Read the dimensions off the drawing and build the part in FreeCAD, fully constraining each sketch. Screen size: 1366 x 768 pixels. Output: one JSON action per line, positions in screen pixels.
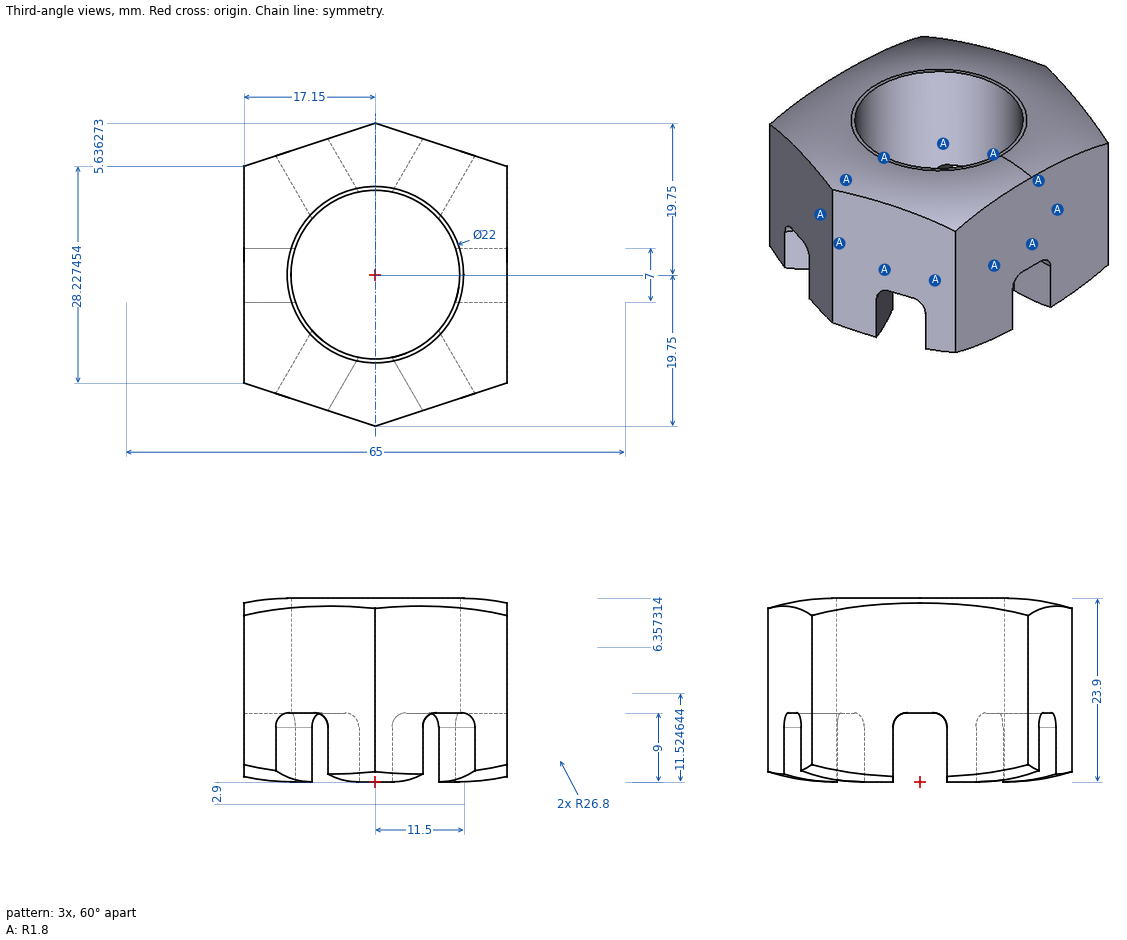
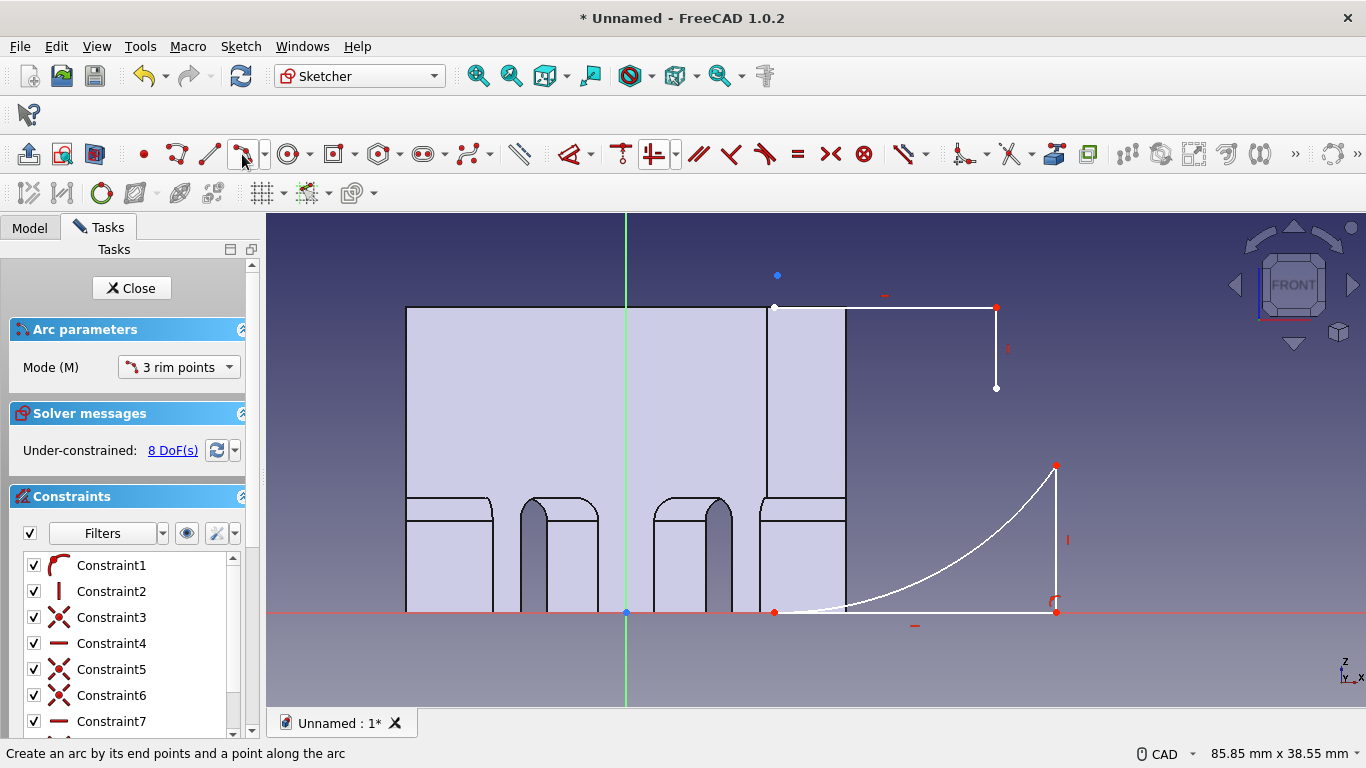
{"action": "left_click", "coordinate": [996, 389]}
{"action": "left_click", "coordinate": [774, 308]}
{"action": "left_click", "coordinate": [892, 328]}
{"action": "key", "text": "Escape"}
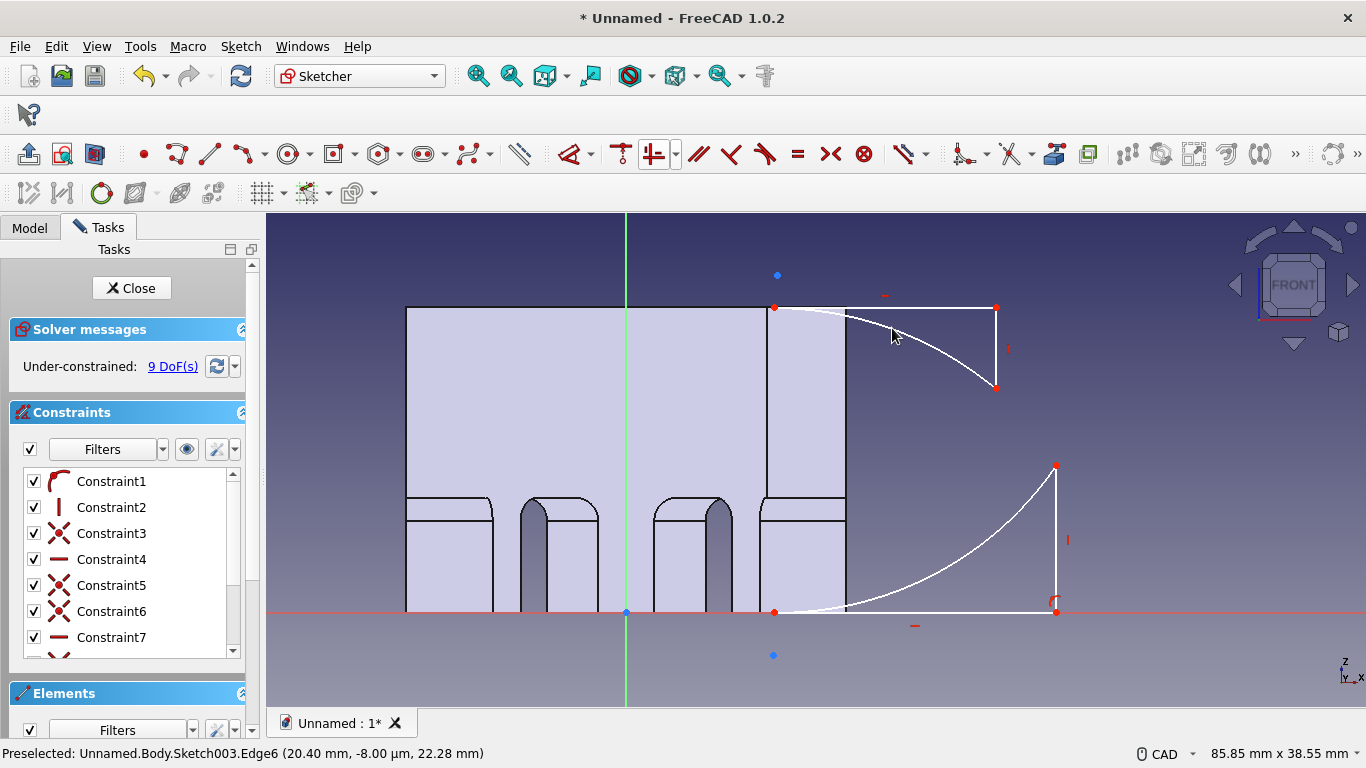
{"action": "left_click", "coordinate": [971, 613]}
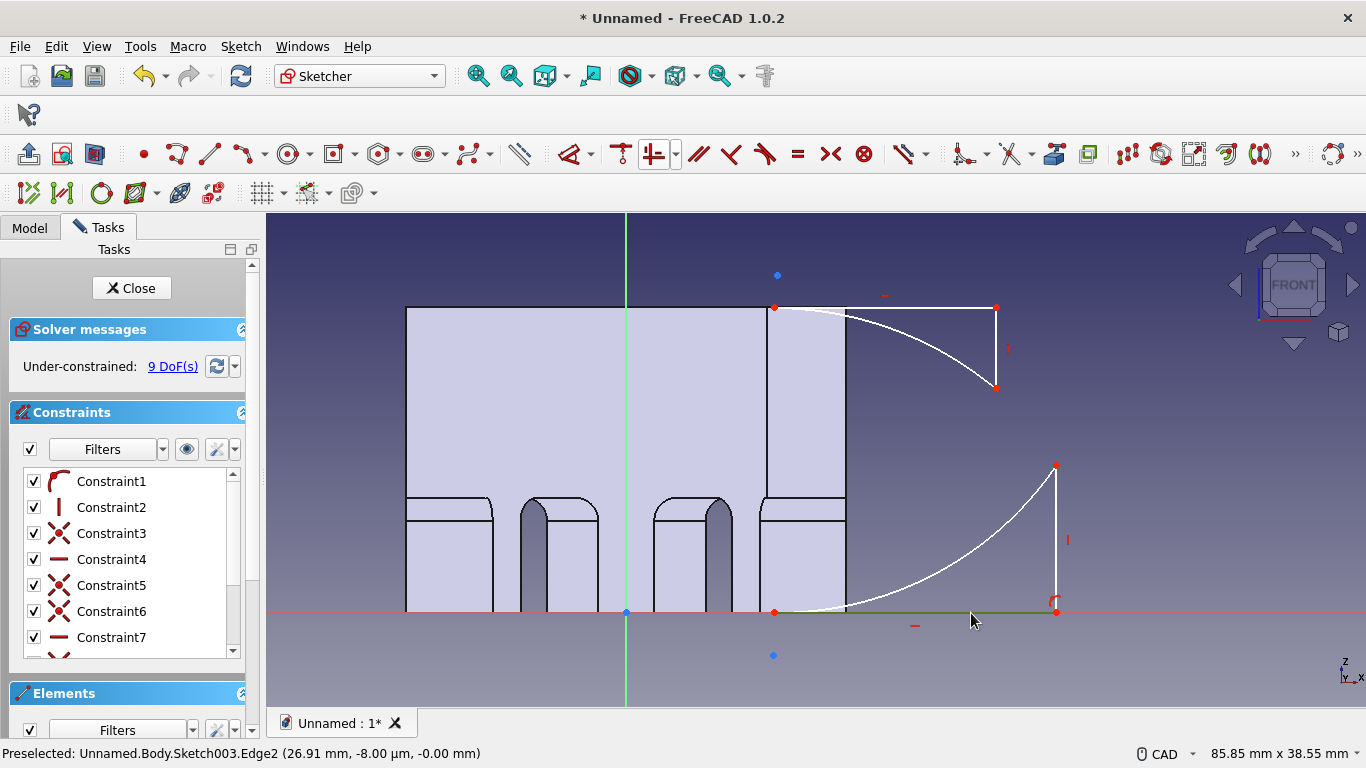
{"action": "left_click", "coordinate": [872, 599]}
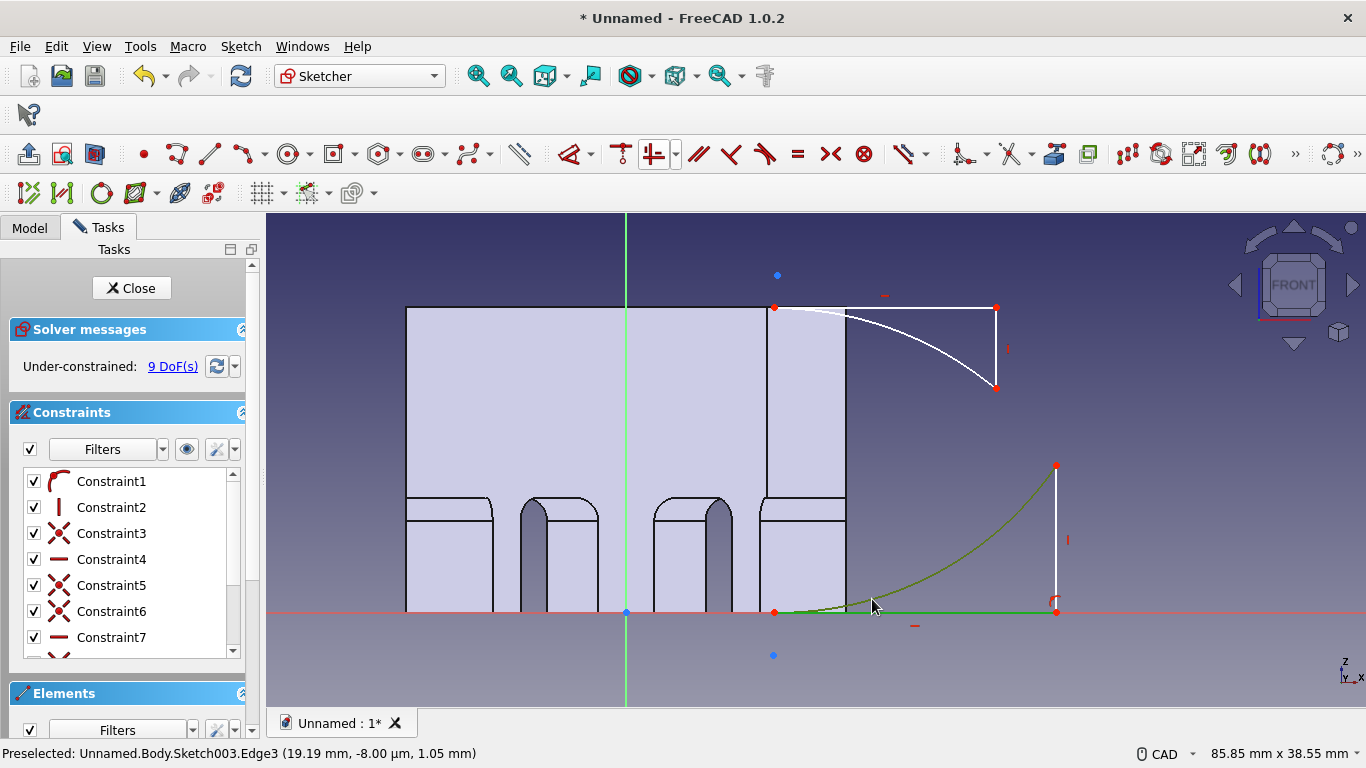
{"action": "left_click", "coordinate": [765, 154]}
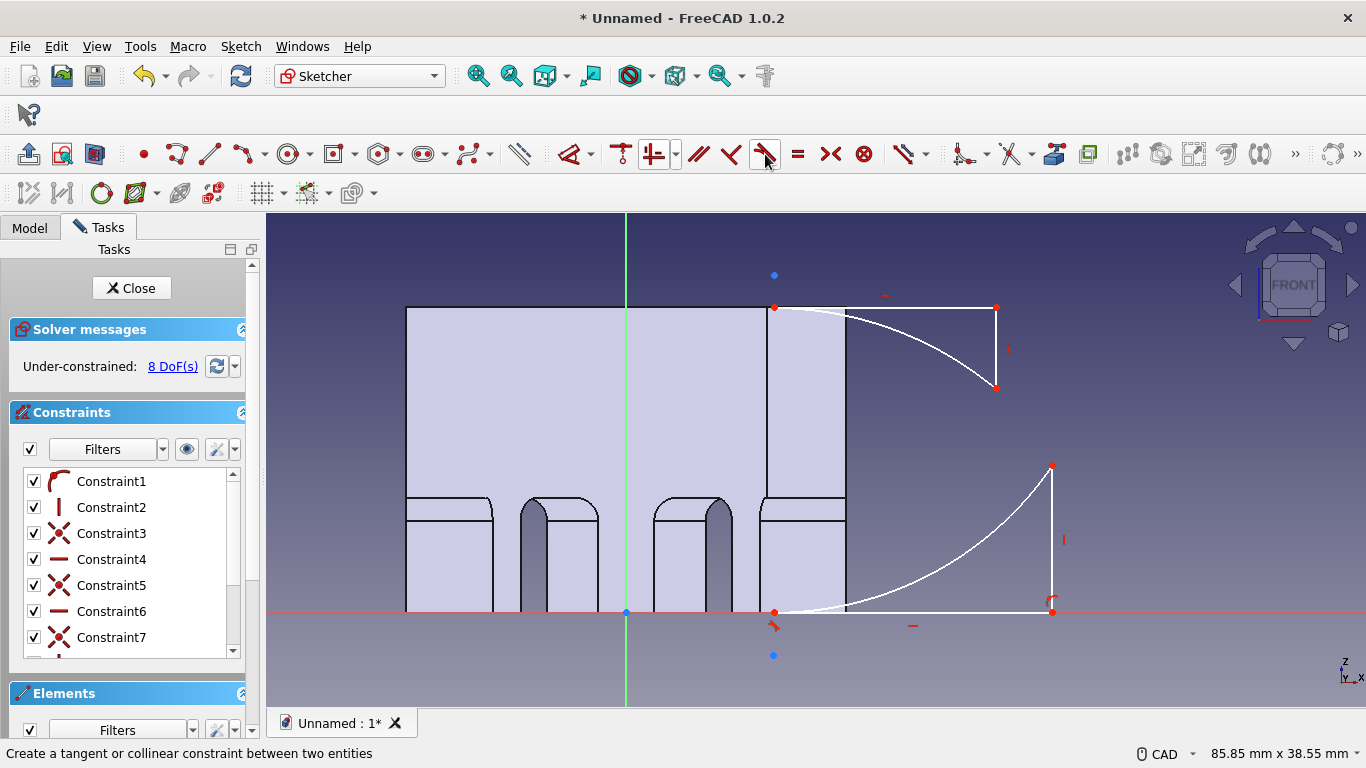
{"action": "left_click", "coordinate": [929, 308]}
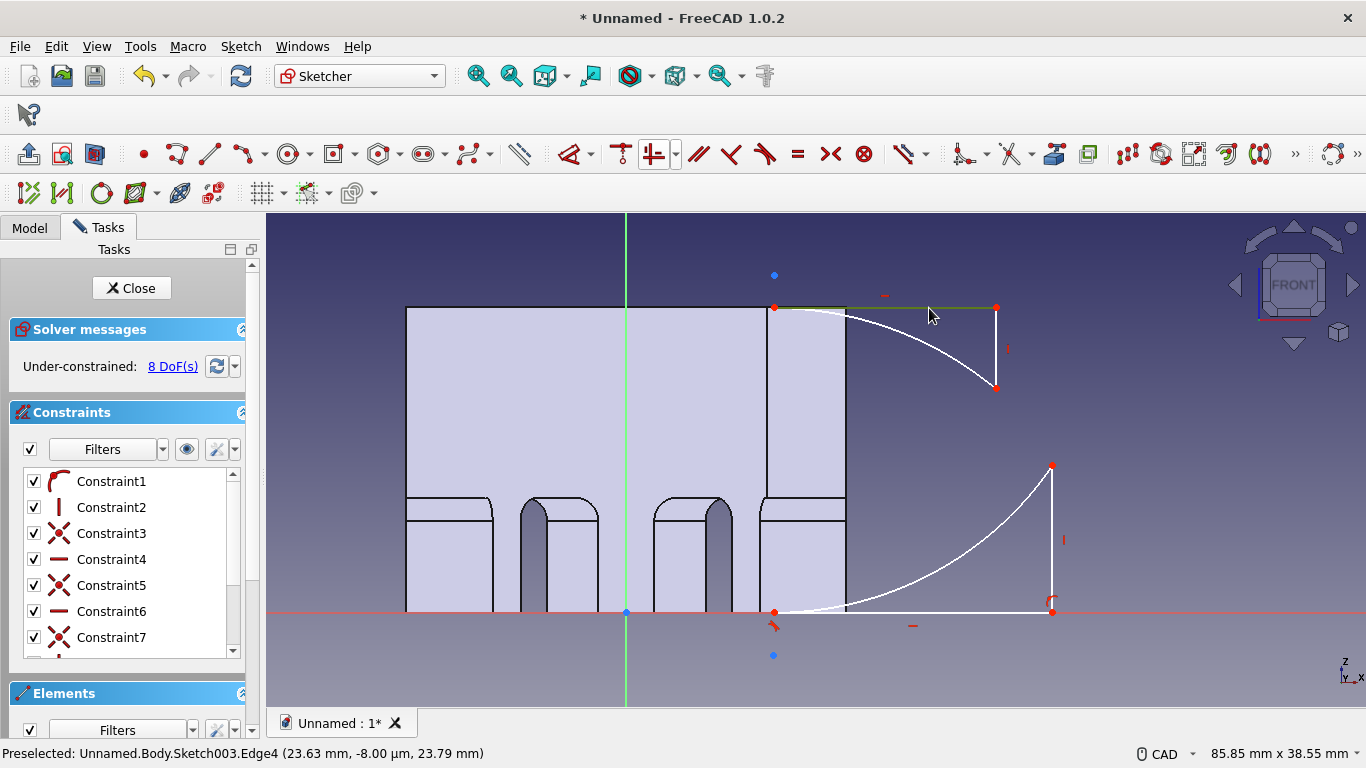
{"action": "left_click", "coordinate": [936, 349]}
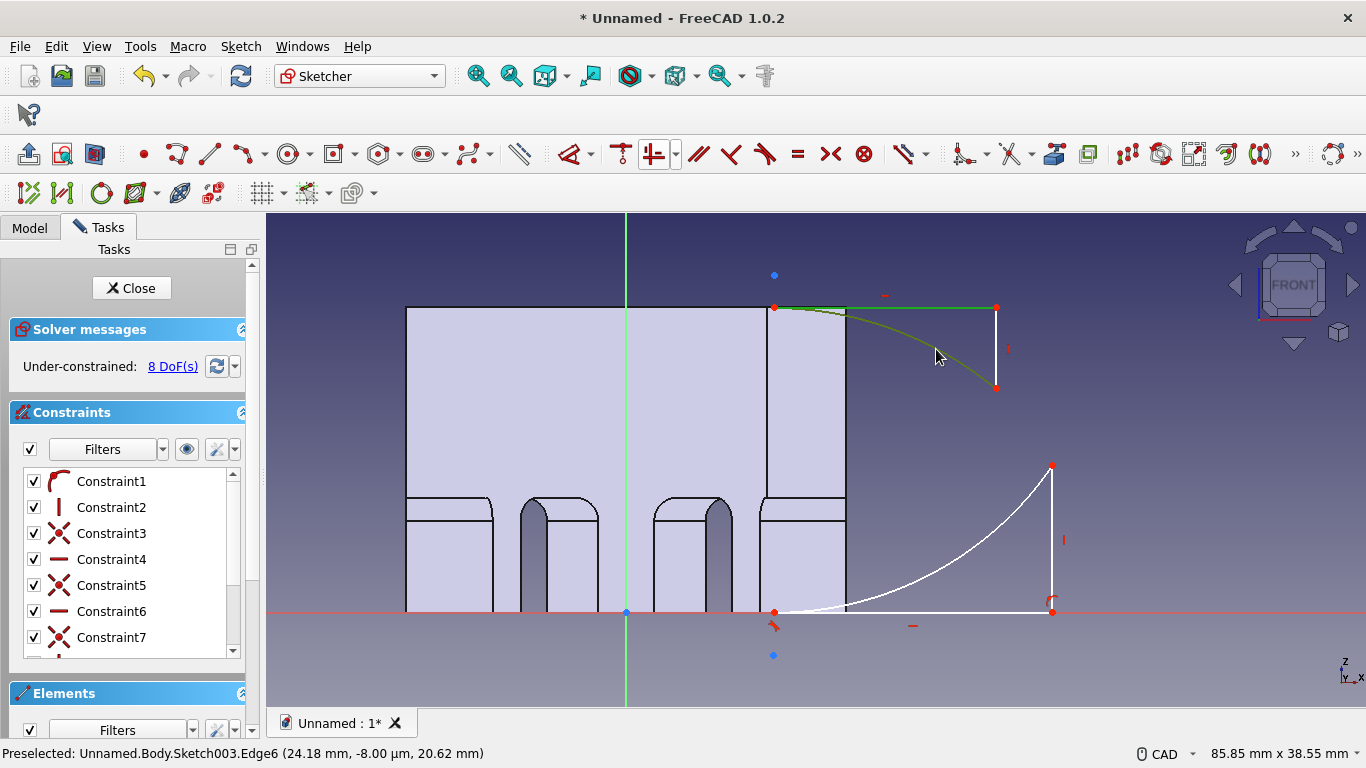
{"action": "left_click", "coordinate": [765, 154]}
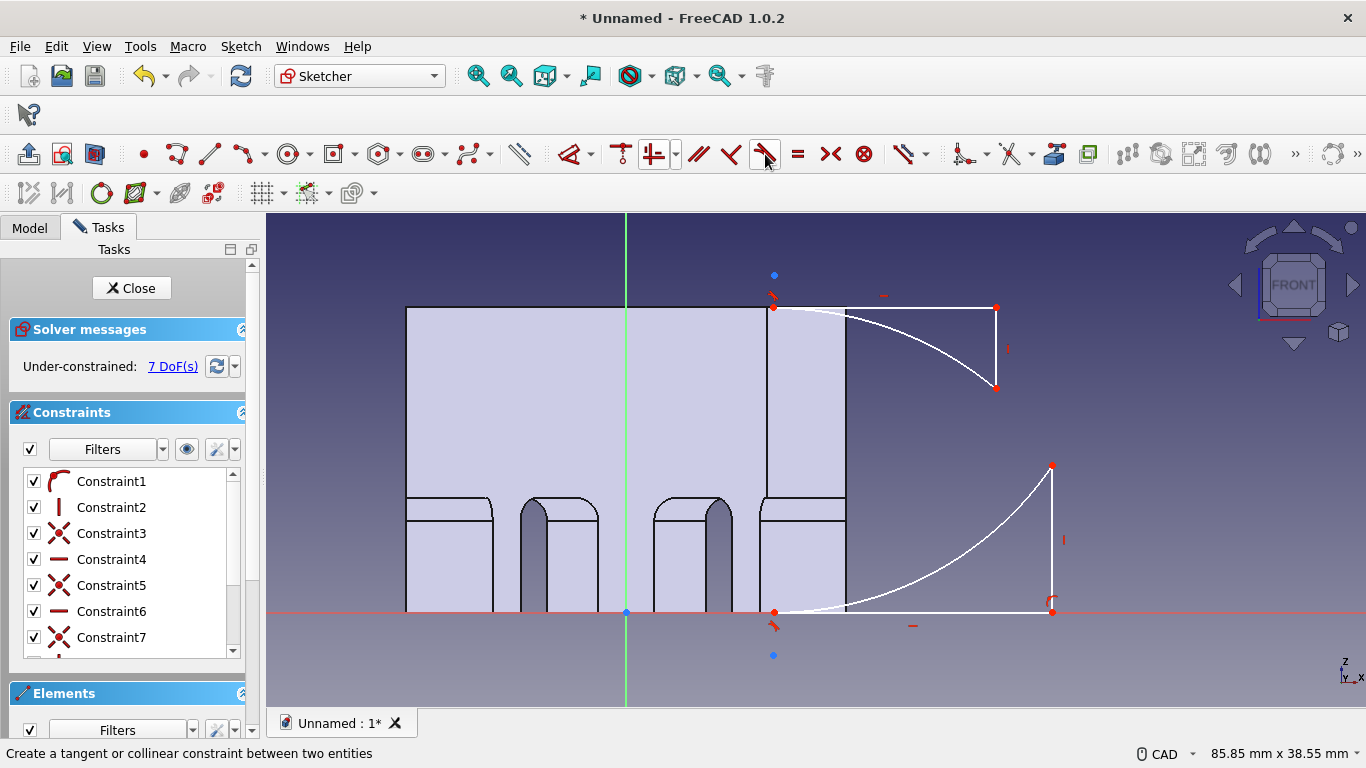
{"action": "left_click", "coordinate": [871, 599]}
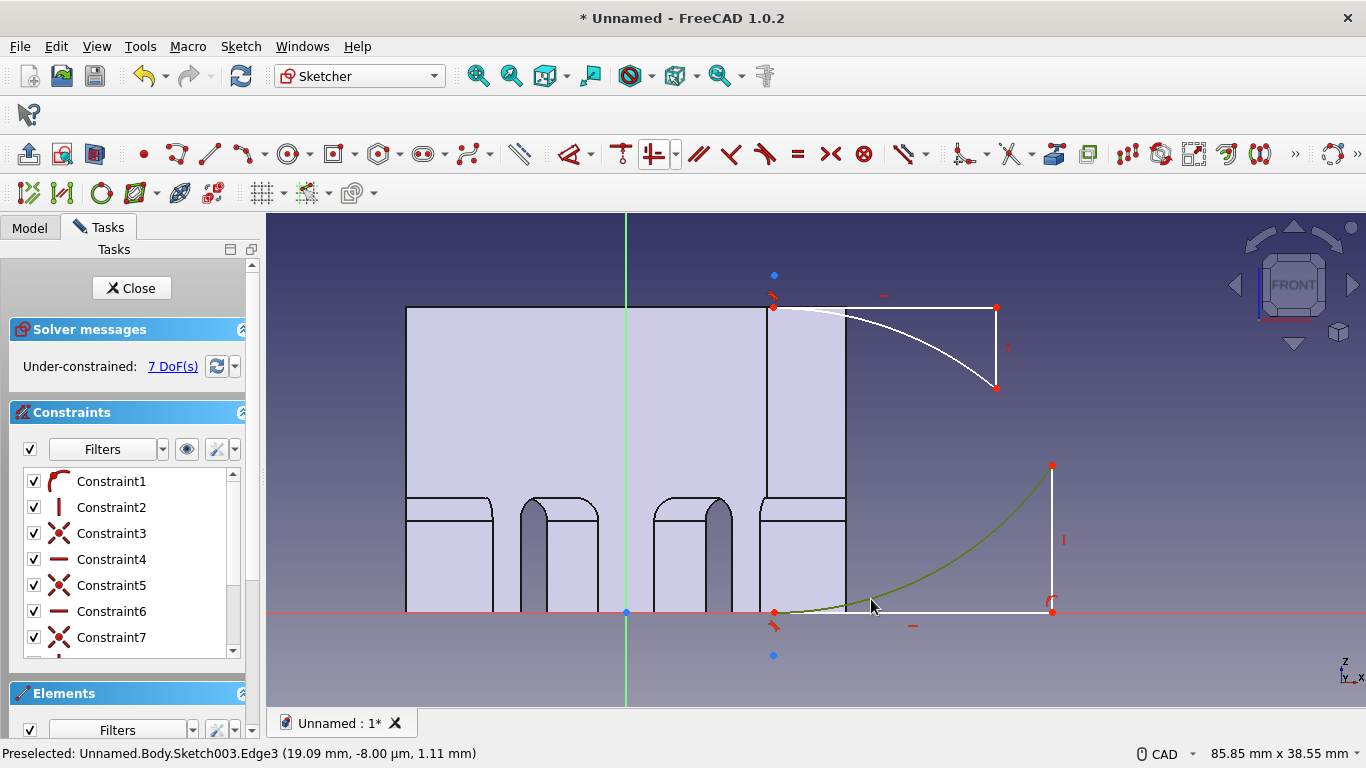
{"action": "left_click", "coordinate": [936, 349]}